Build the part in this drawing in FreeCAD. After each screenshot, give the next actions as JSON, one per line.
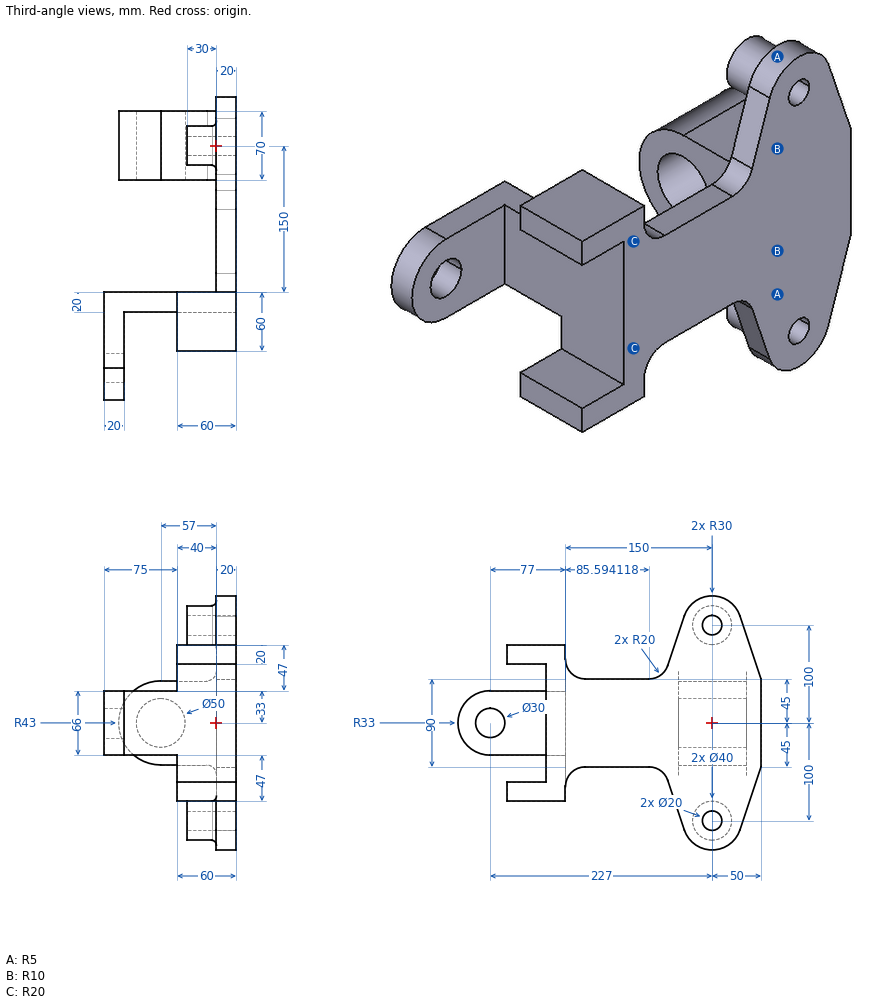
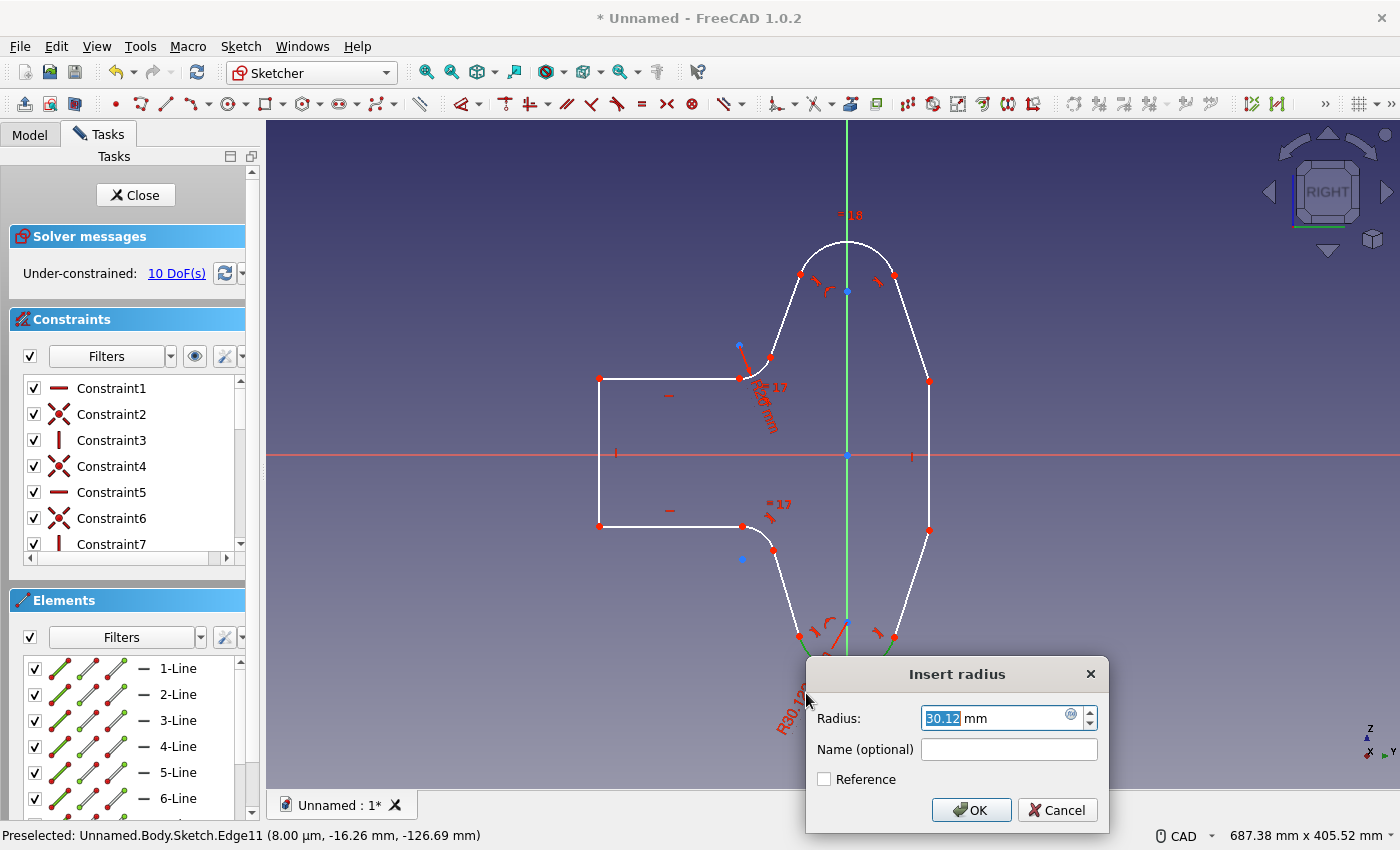
{"action": "type", "text": "30"}
{"action": "key", "text": "Return"}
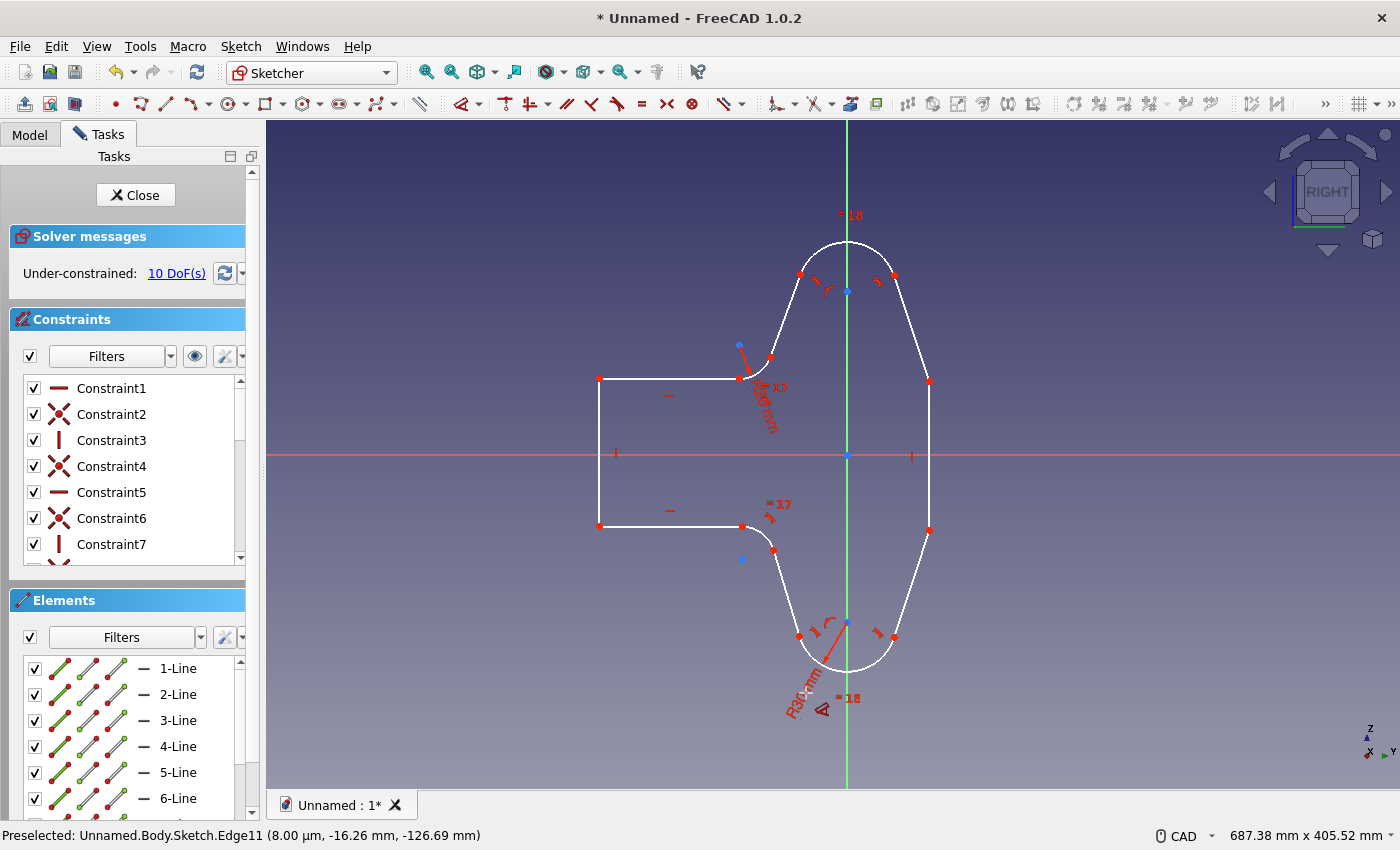
{"action": "left_click", "coordinate": [599, 423]}
{"action": "left_click", "coordinate": [565, 419]}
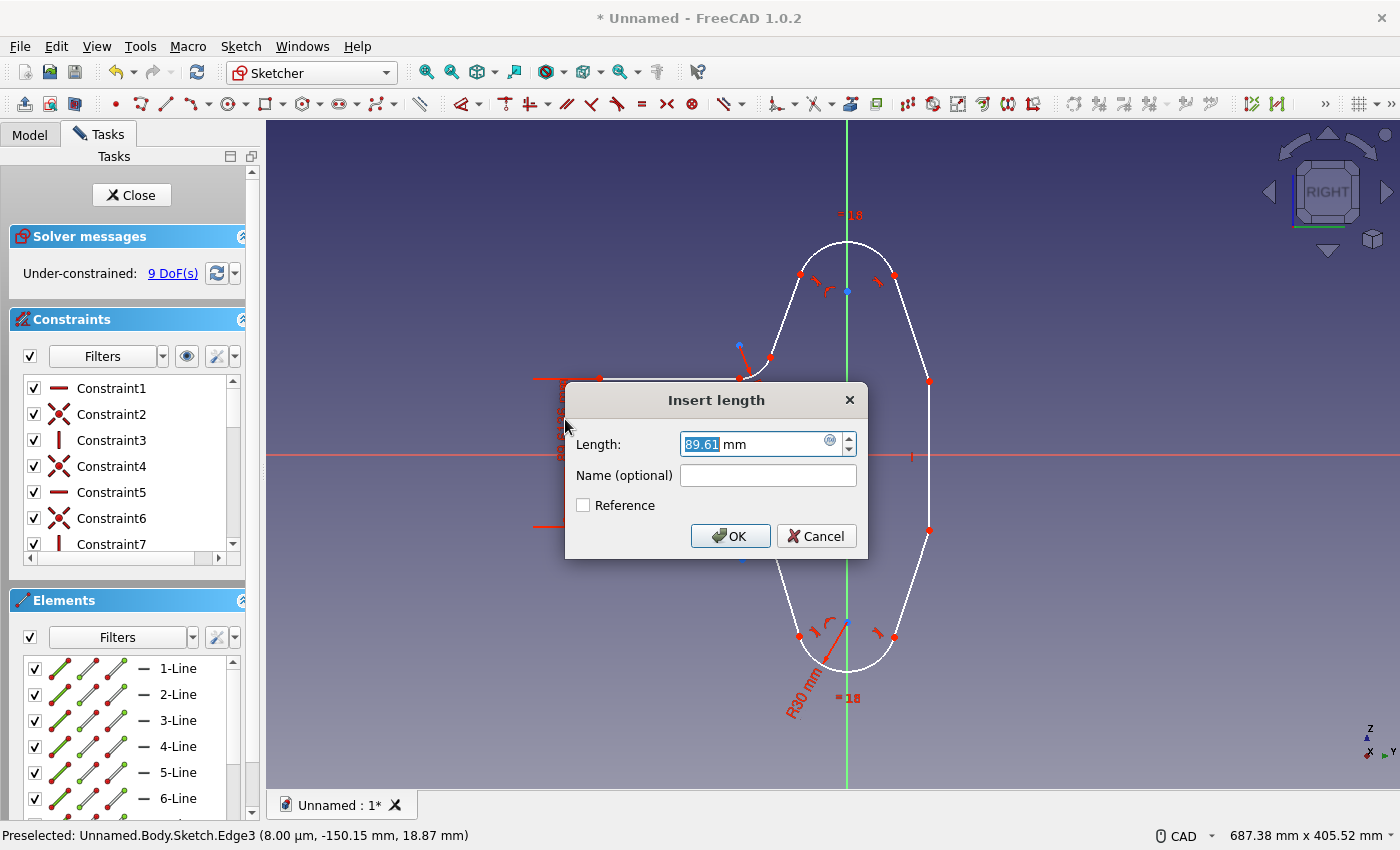
{"action": "type", "text": "90"}
{"action": "key", "text": "Return"}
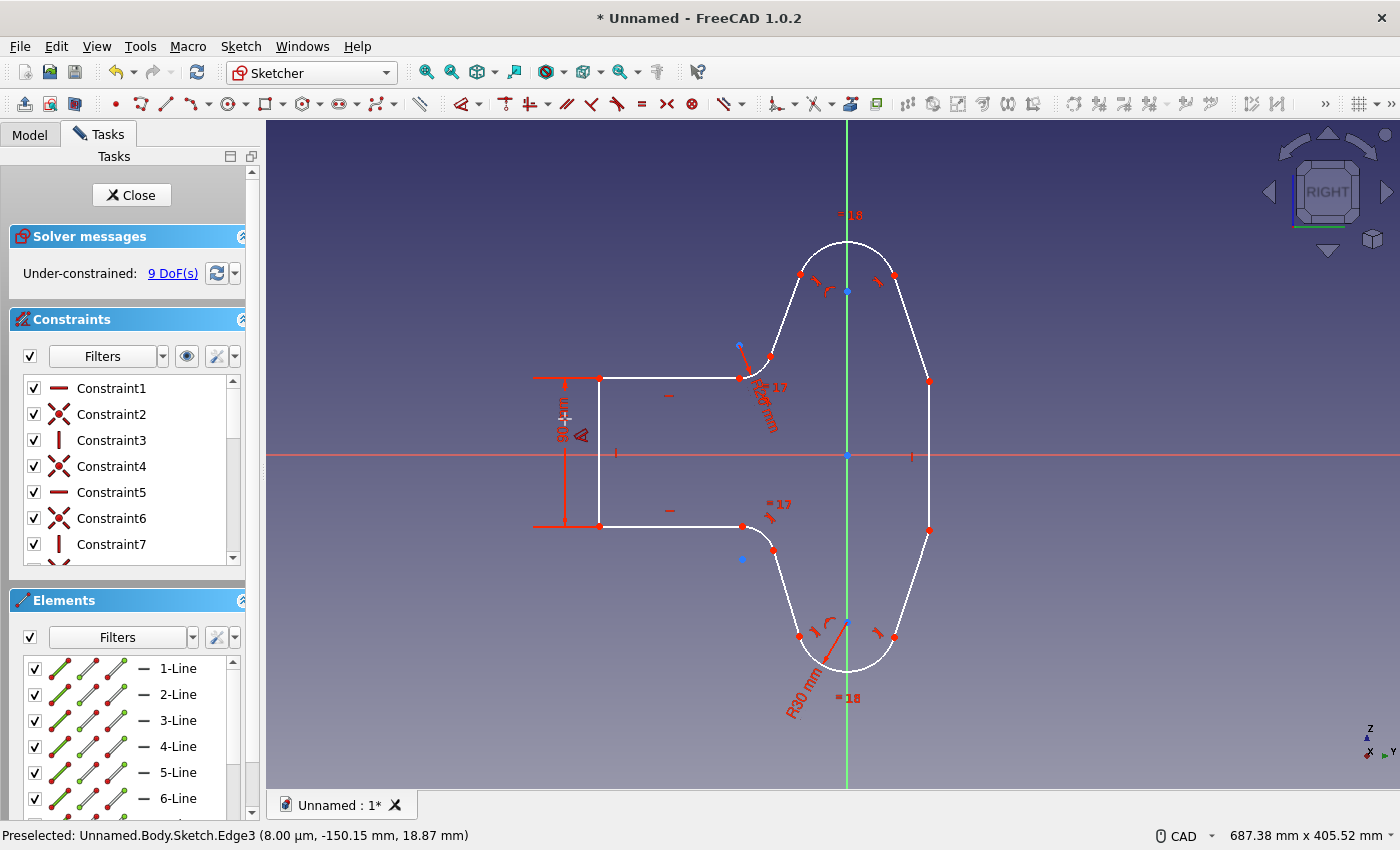
{"action": "left_click", "coordinate": [929, 486]}
{"action": "left_click", "coordinate": [963, 422]}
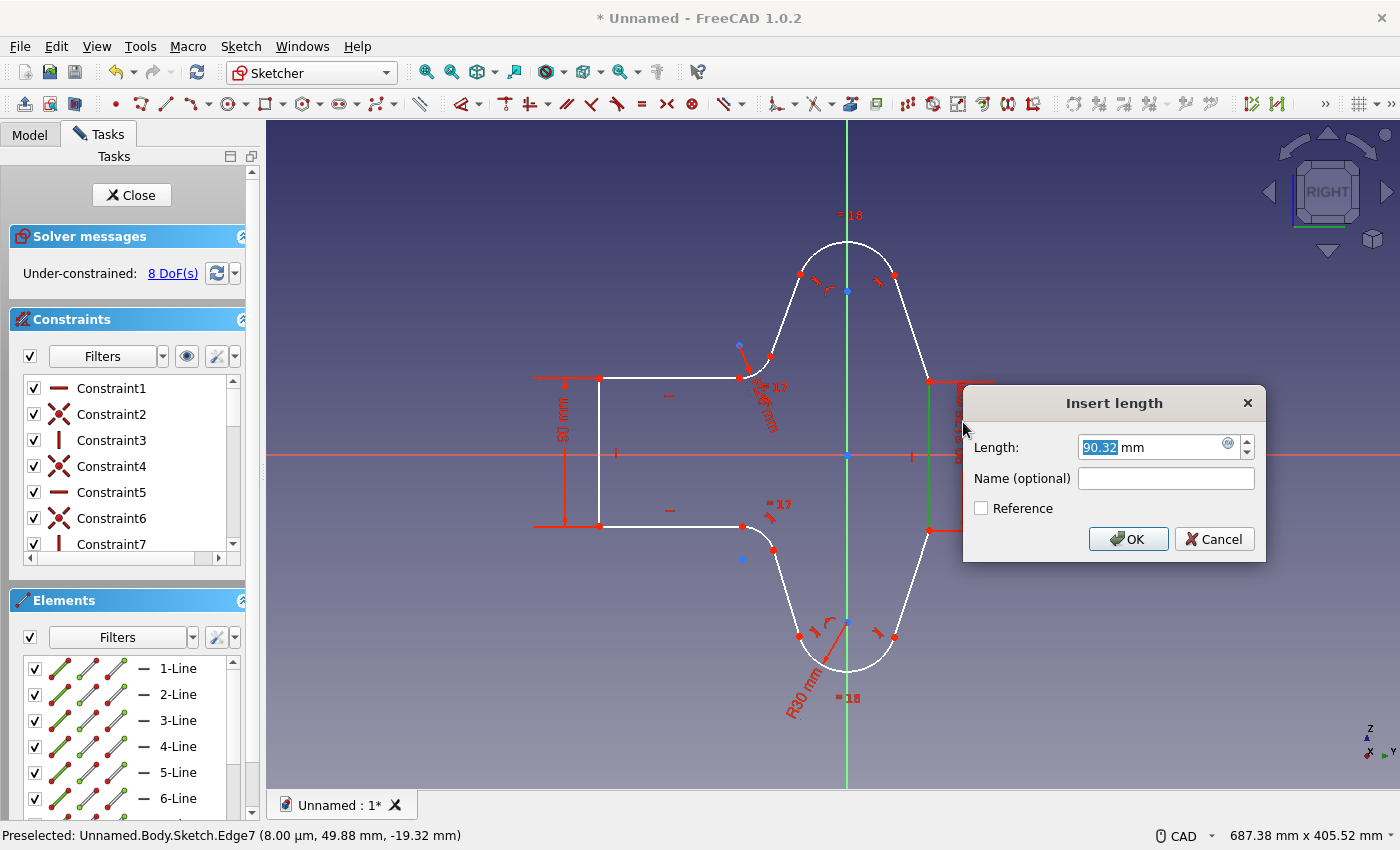
{"action": "type", "text": "90"}
{"action": "key", "text": "Return"}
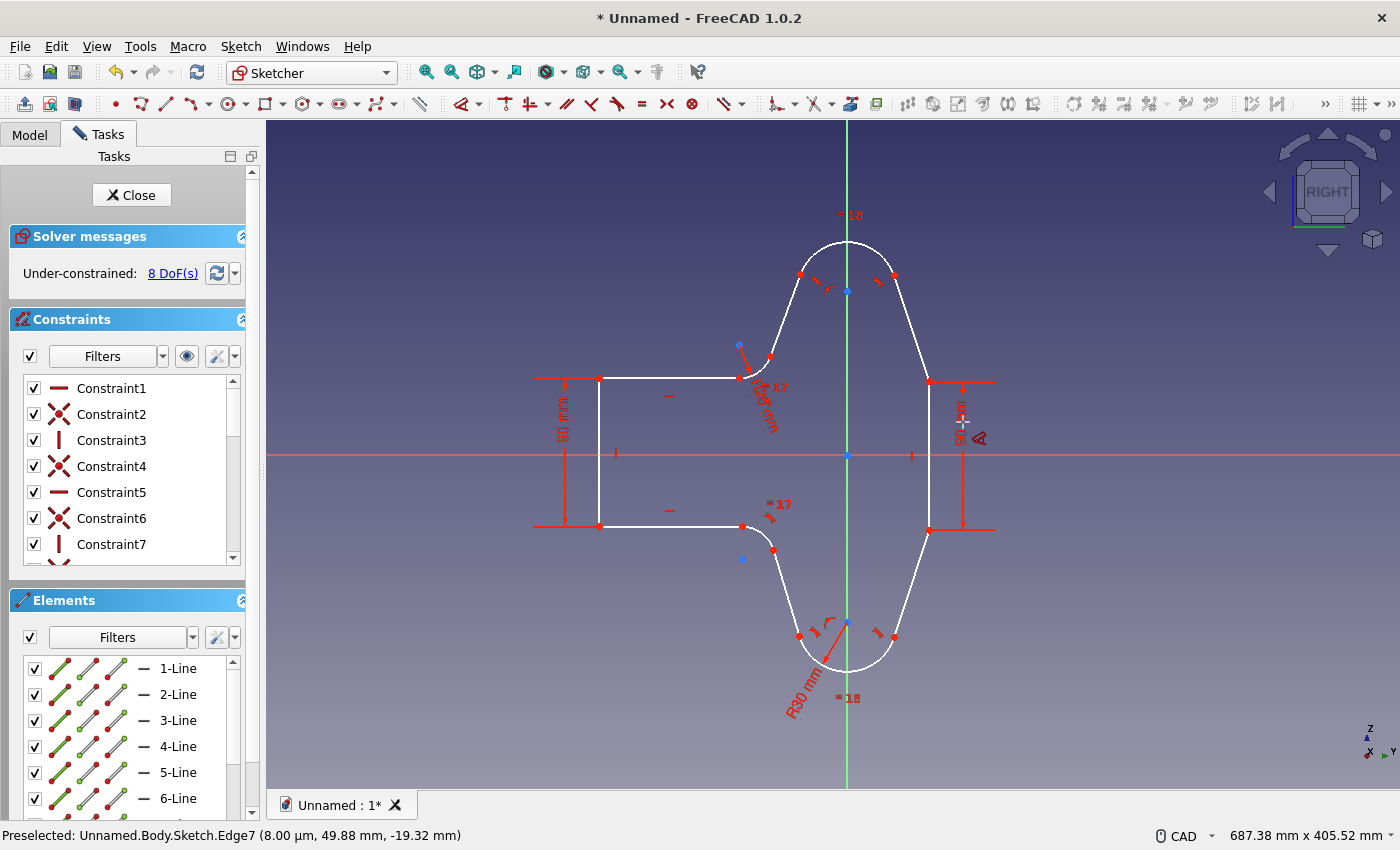
{"action": "left_click", "coordinate": [739, 378]}
{"action": "left_click", "coordinate": [881, 417]}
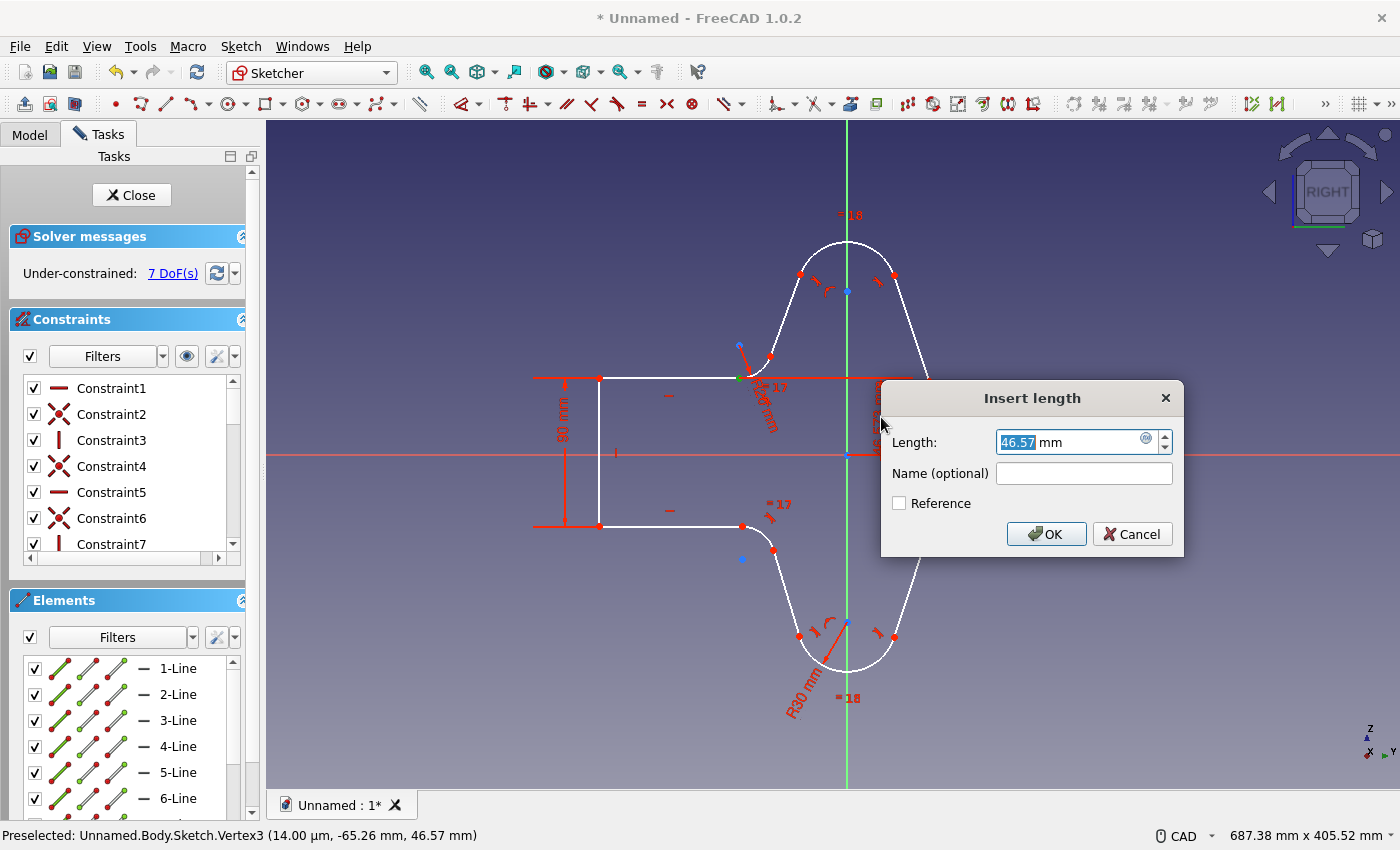
{"action": "type", "text": "45"}
{"action": "key", "text": "Return"}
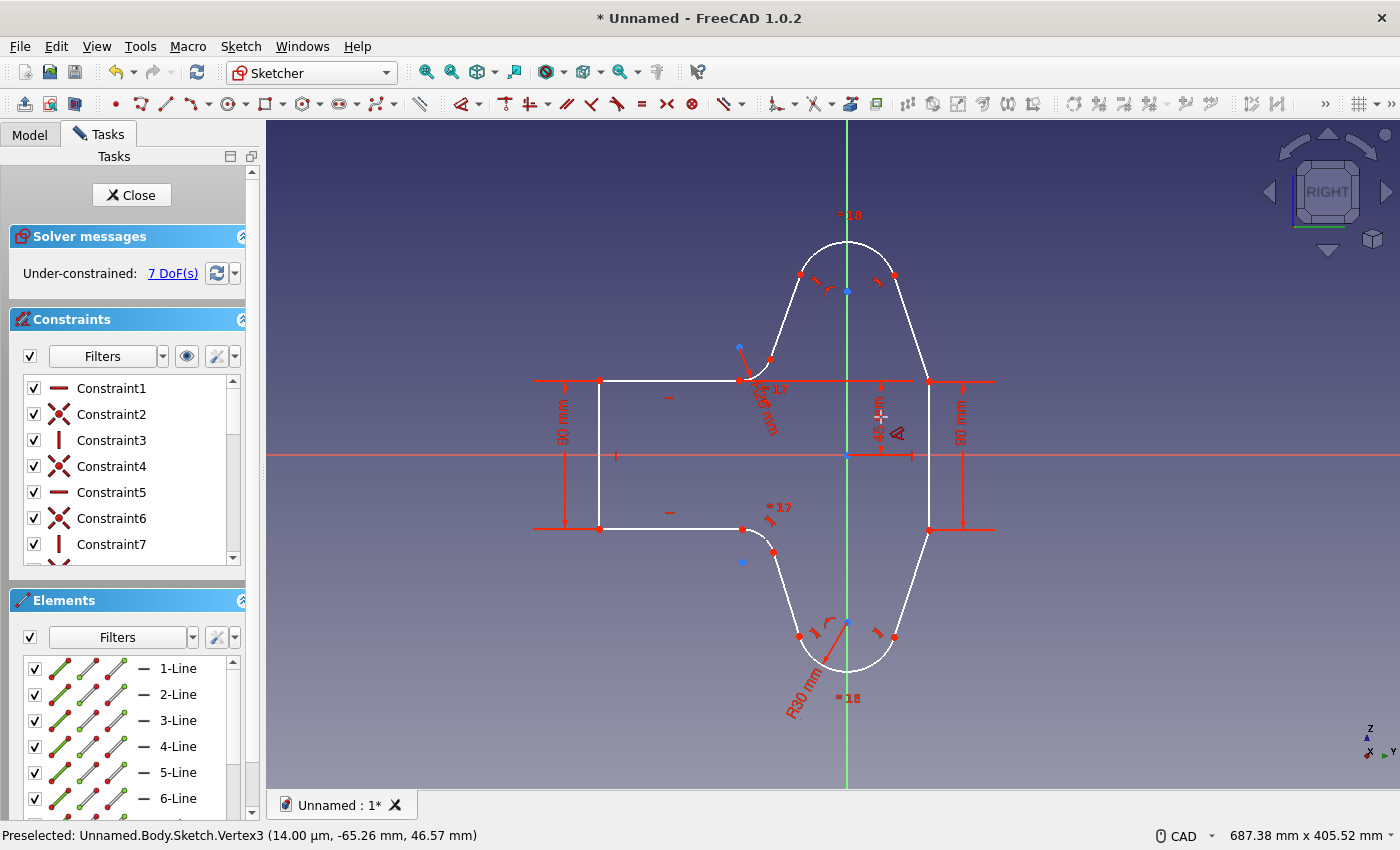
{"action": "left_click", "coordinate": [929, 530]}
{"action": "left_click", "coordinate": [888, 564]}